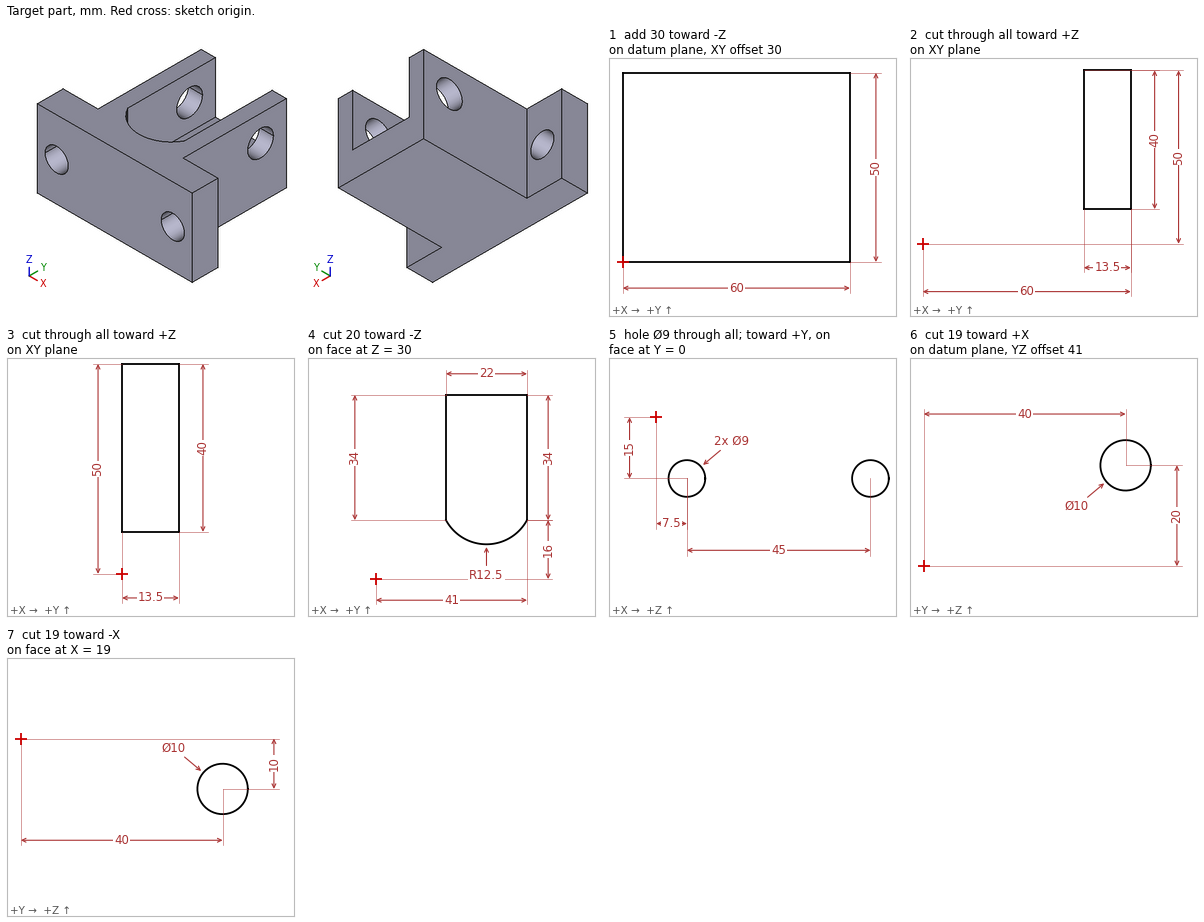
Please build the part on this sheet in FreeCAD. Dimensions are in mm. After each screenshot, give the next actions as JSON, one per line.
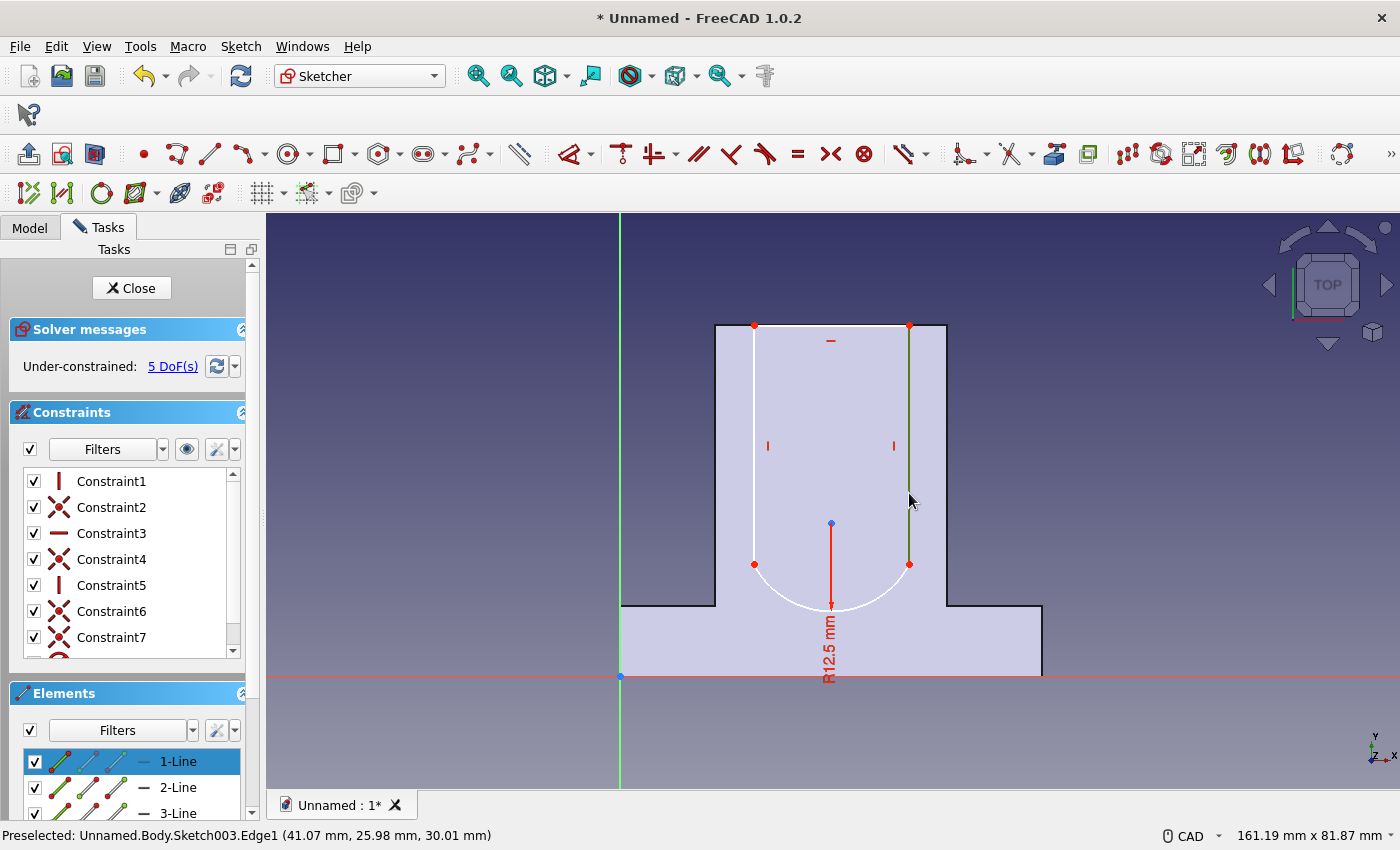
{"action": "key", "text": "i"}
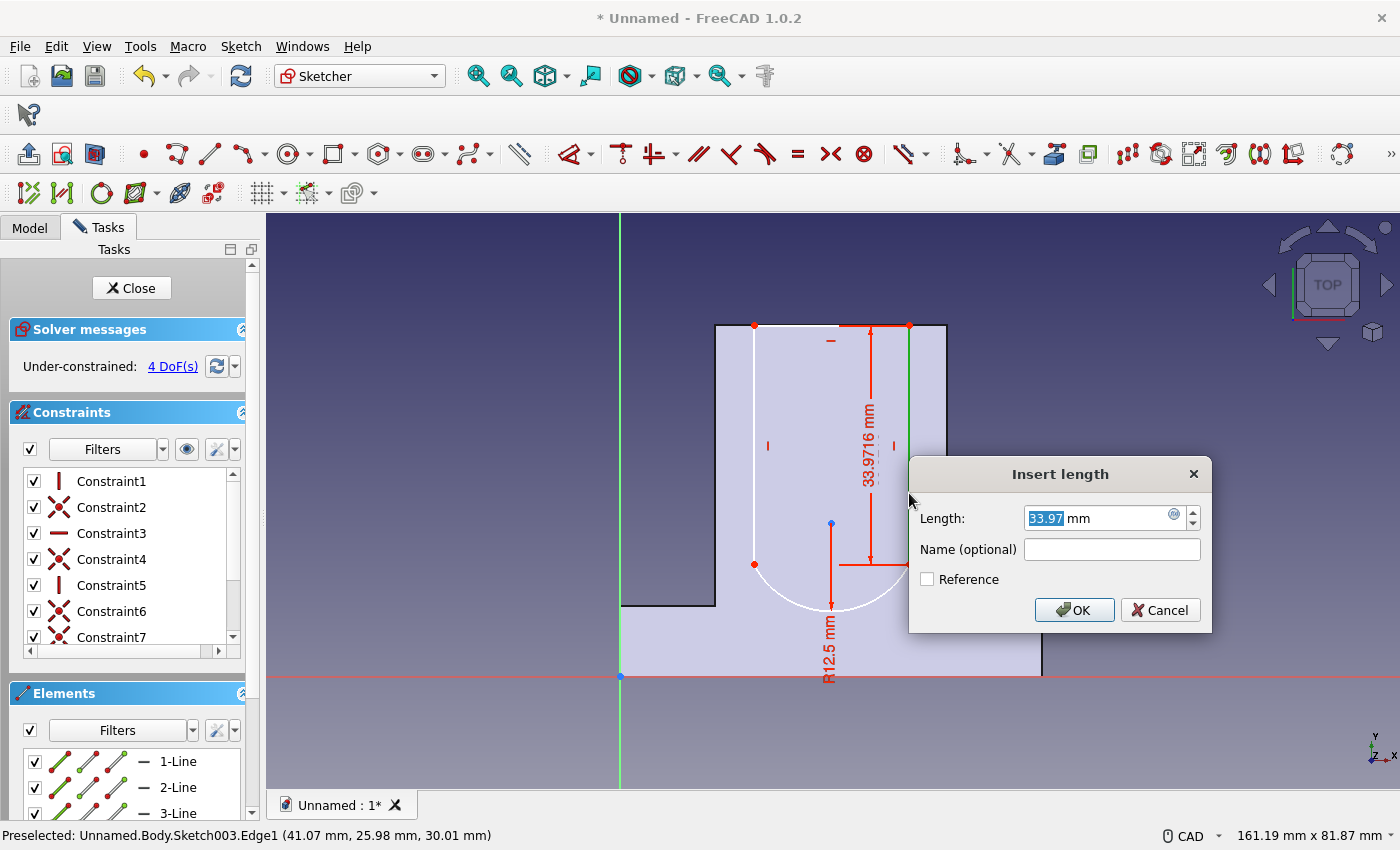
{"action": "type", "text": "34"}
{"action": "key", "text": "Return"}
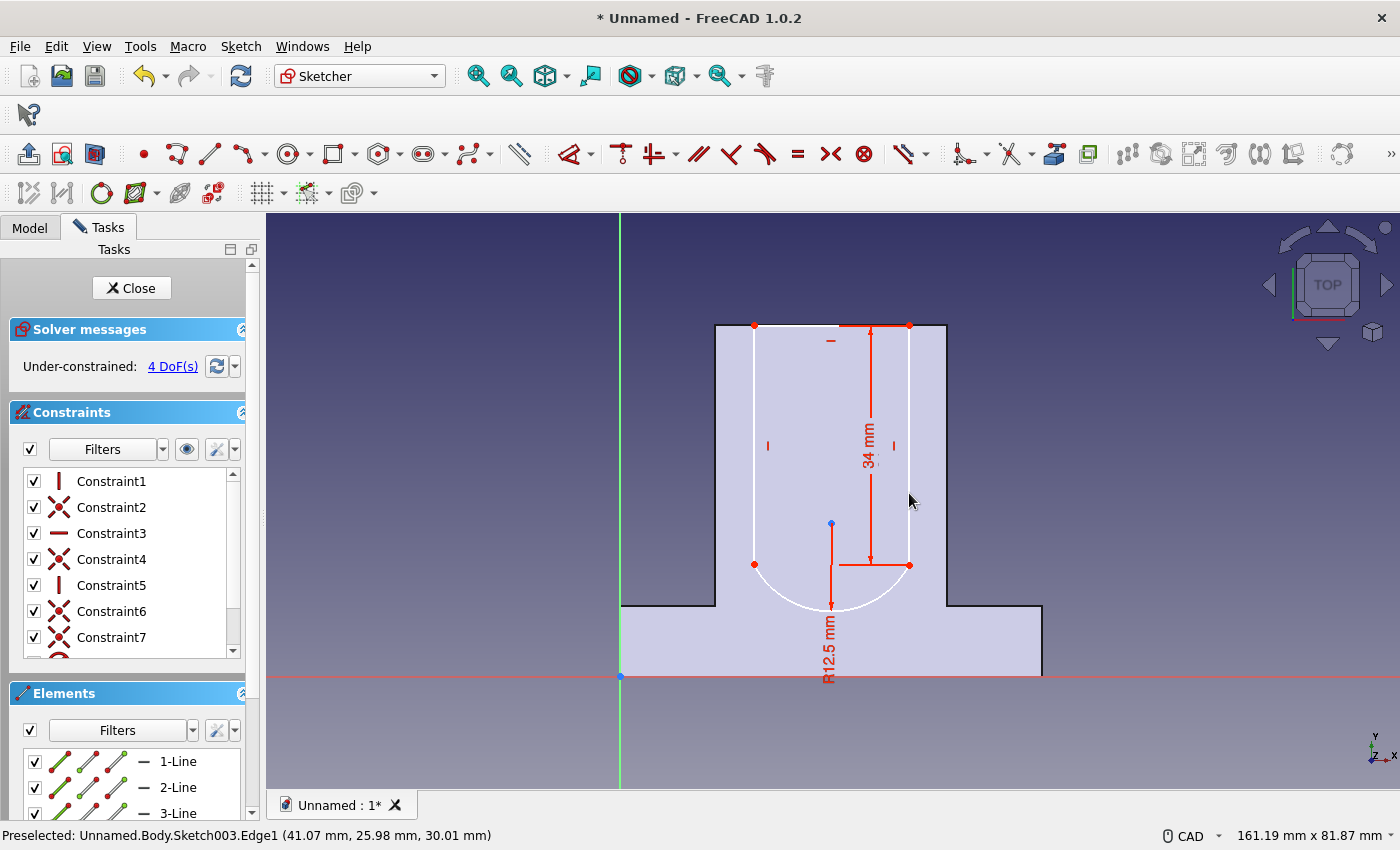
{"action": "left_click", "coordinate": [862, 326]}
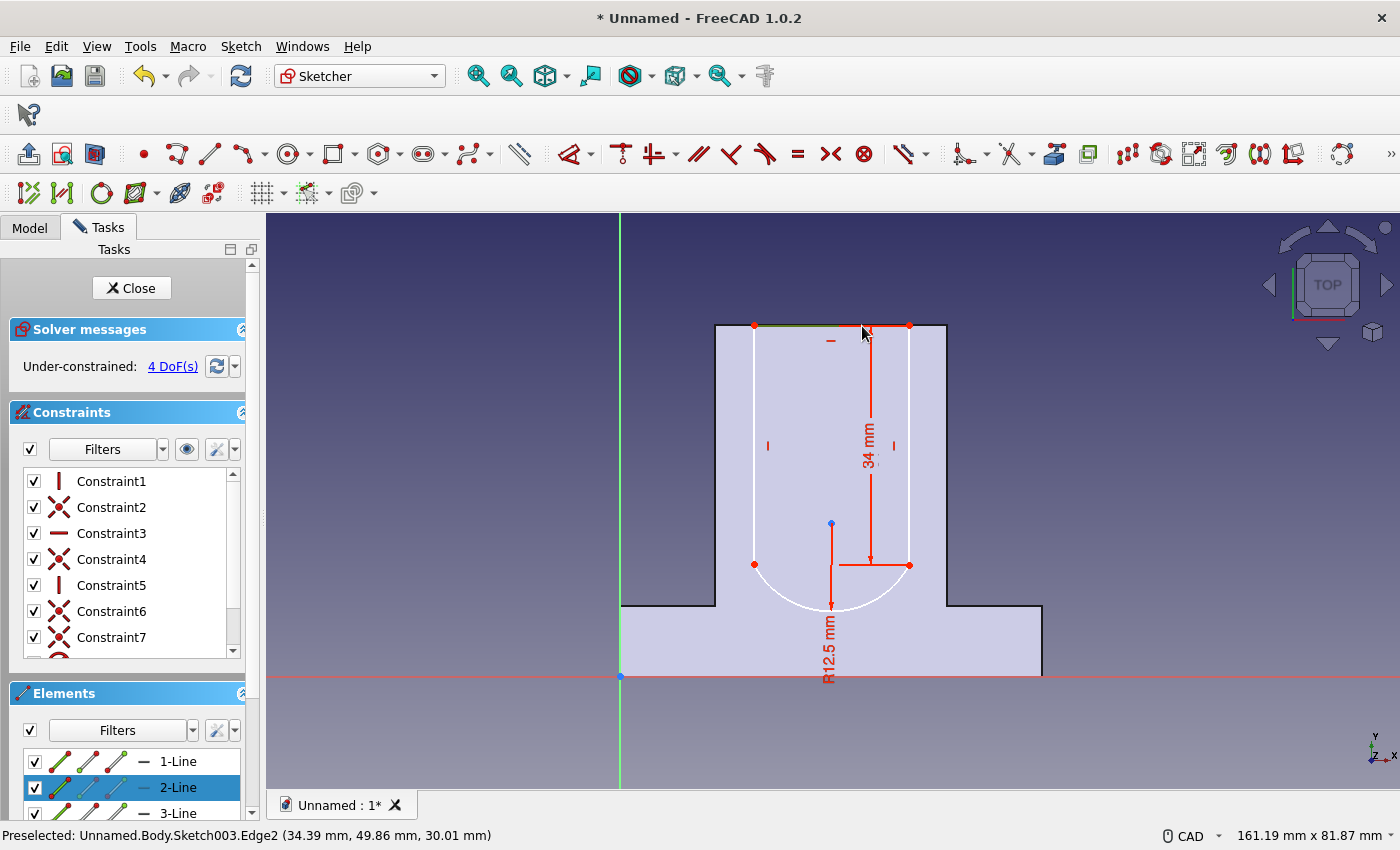
{"action": "key", "text": "l"}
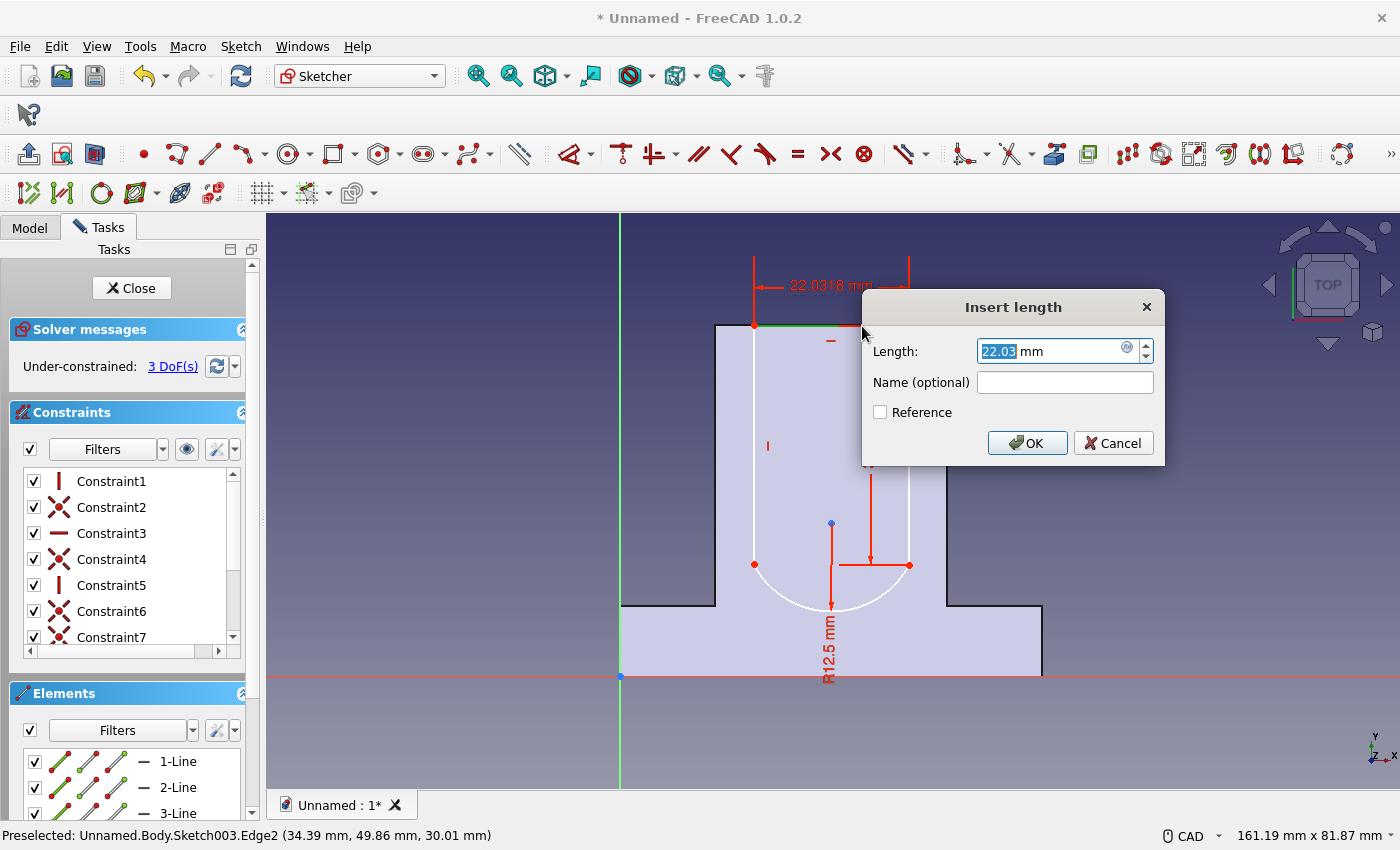
{"action": "type", "text": "22"}
{"action": "key", "text": "Return"}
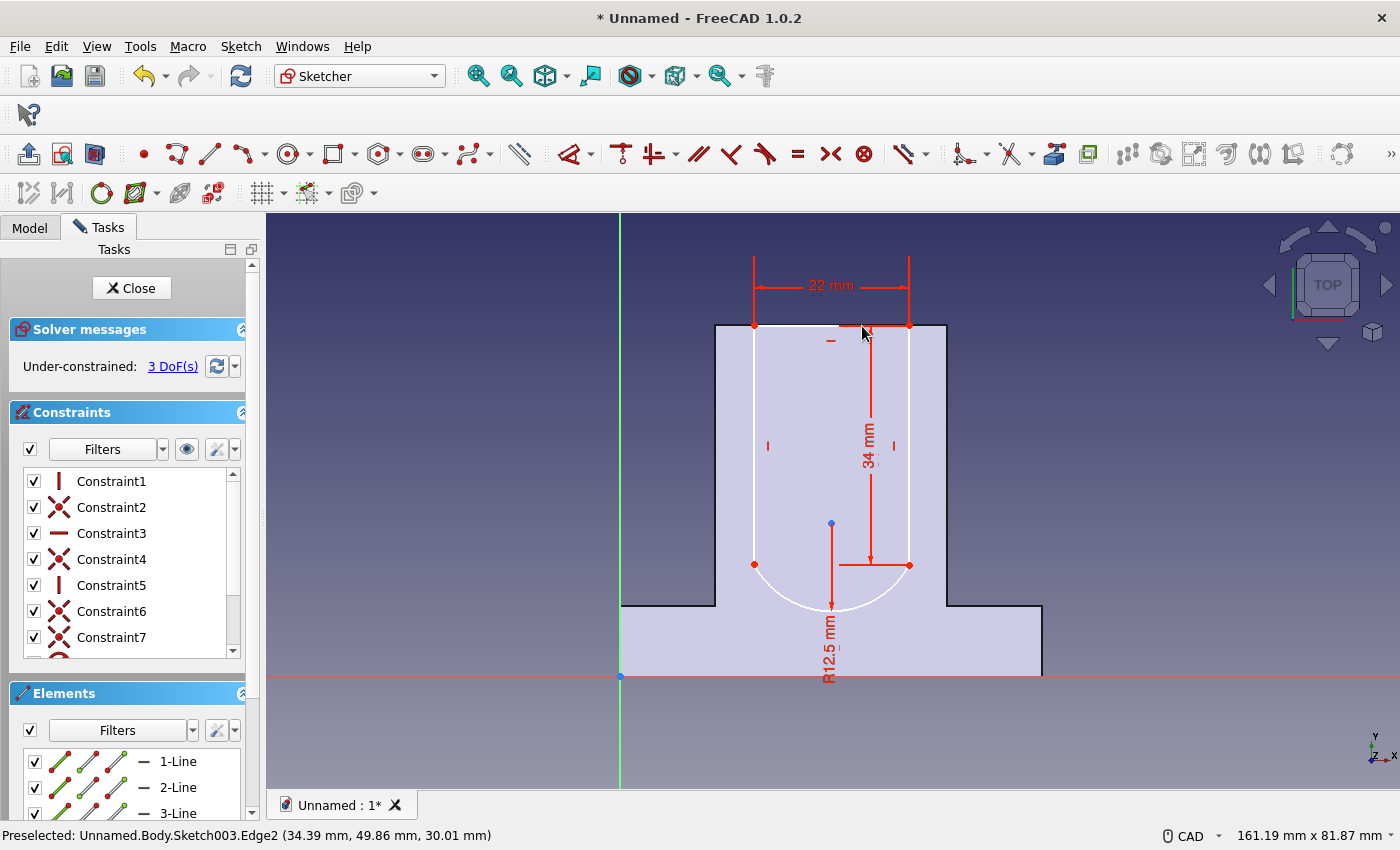
{"action": "left_click", "coordinate": [754, 398]}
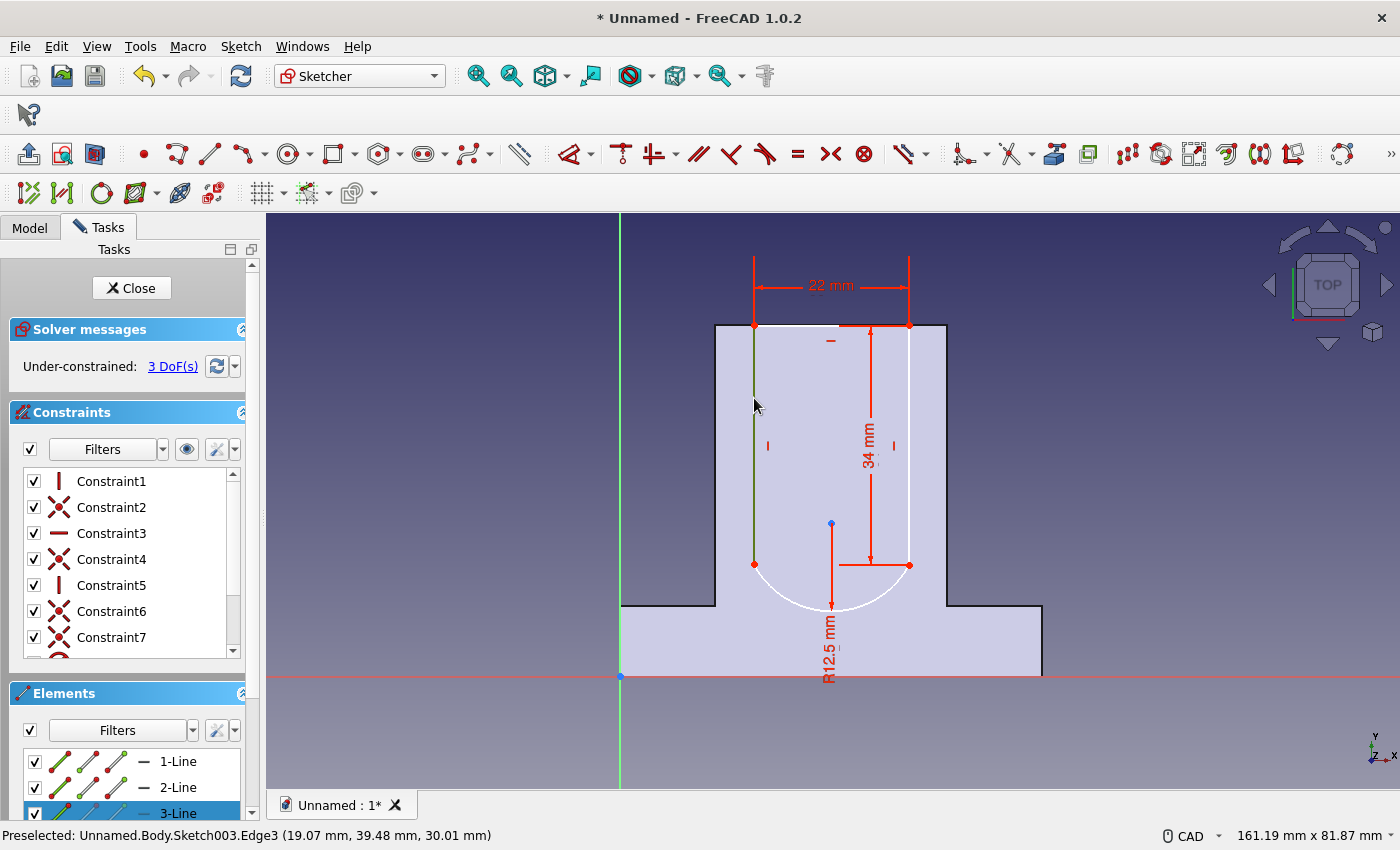
{"action": "key", "text": "i"}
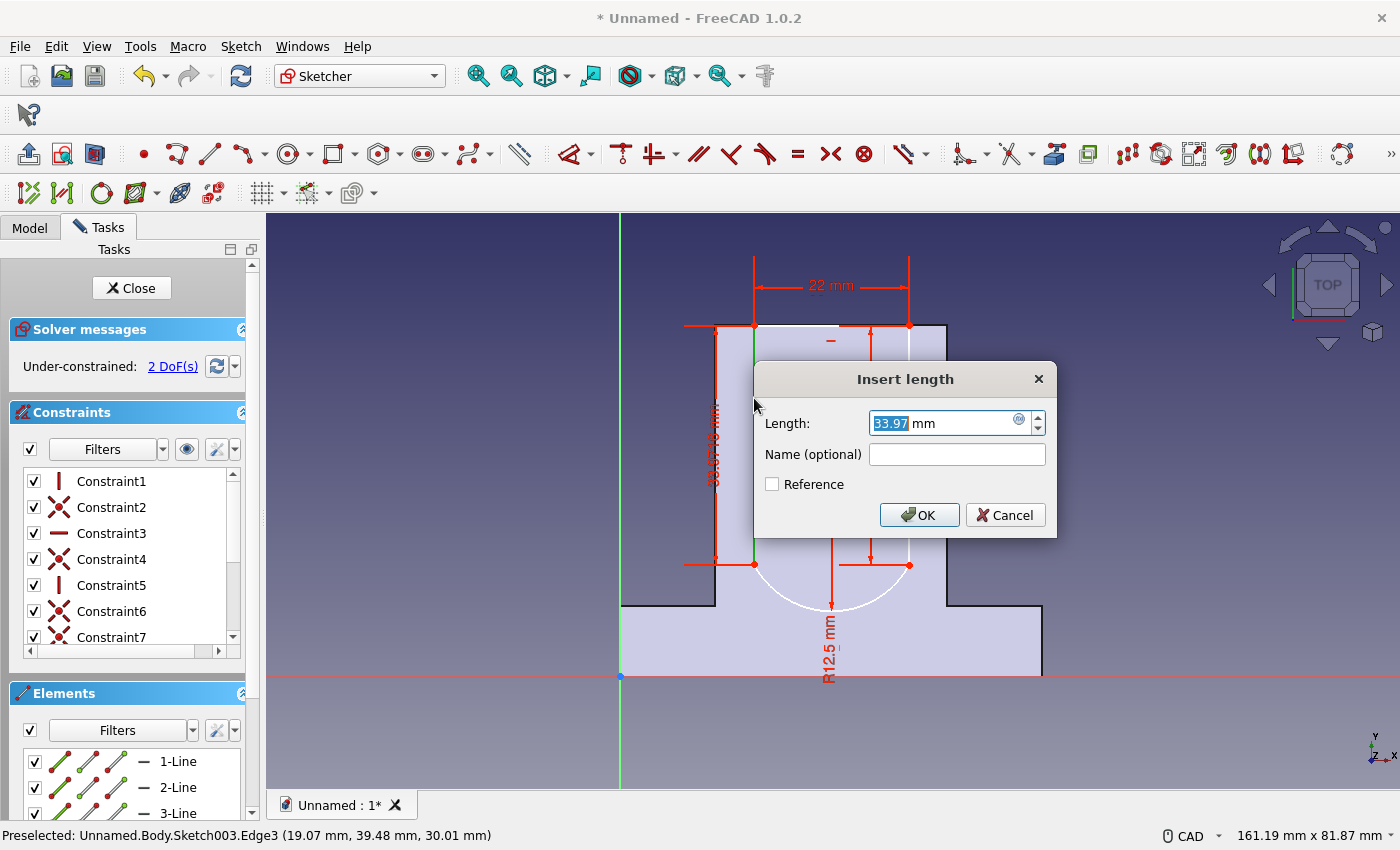
{"action": "type", "text": "34"}
{"action": "key", "text": "Return"}